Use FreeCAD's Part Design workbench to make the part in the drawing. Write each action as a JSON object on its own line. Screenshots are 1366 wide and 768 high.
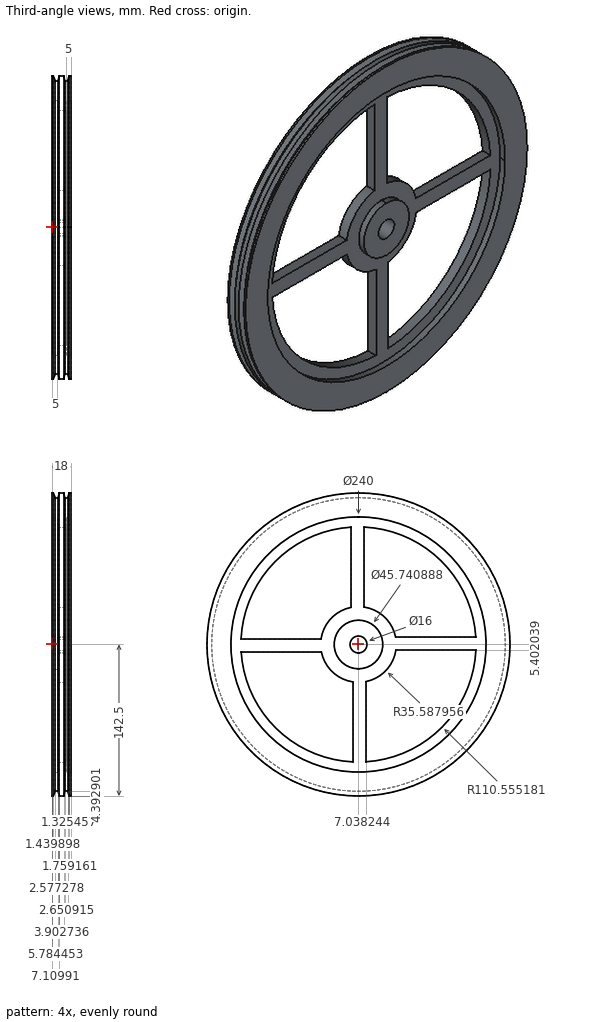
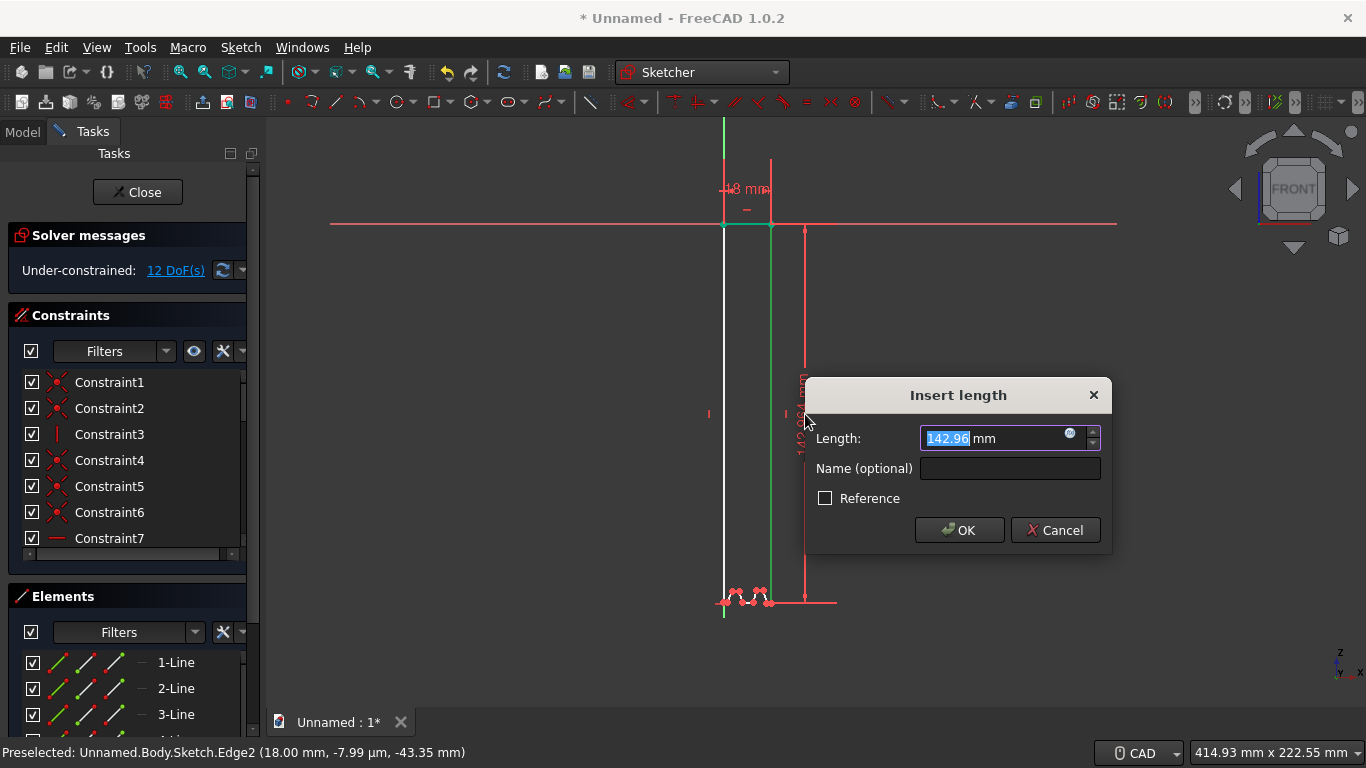
{"action": "type", "text": "142.5"}
{"action": "key", "text": "Return"}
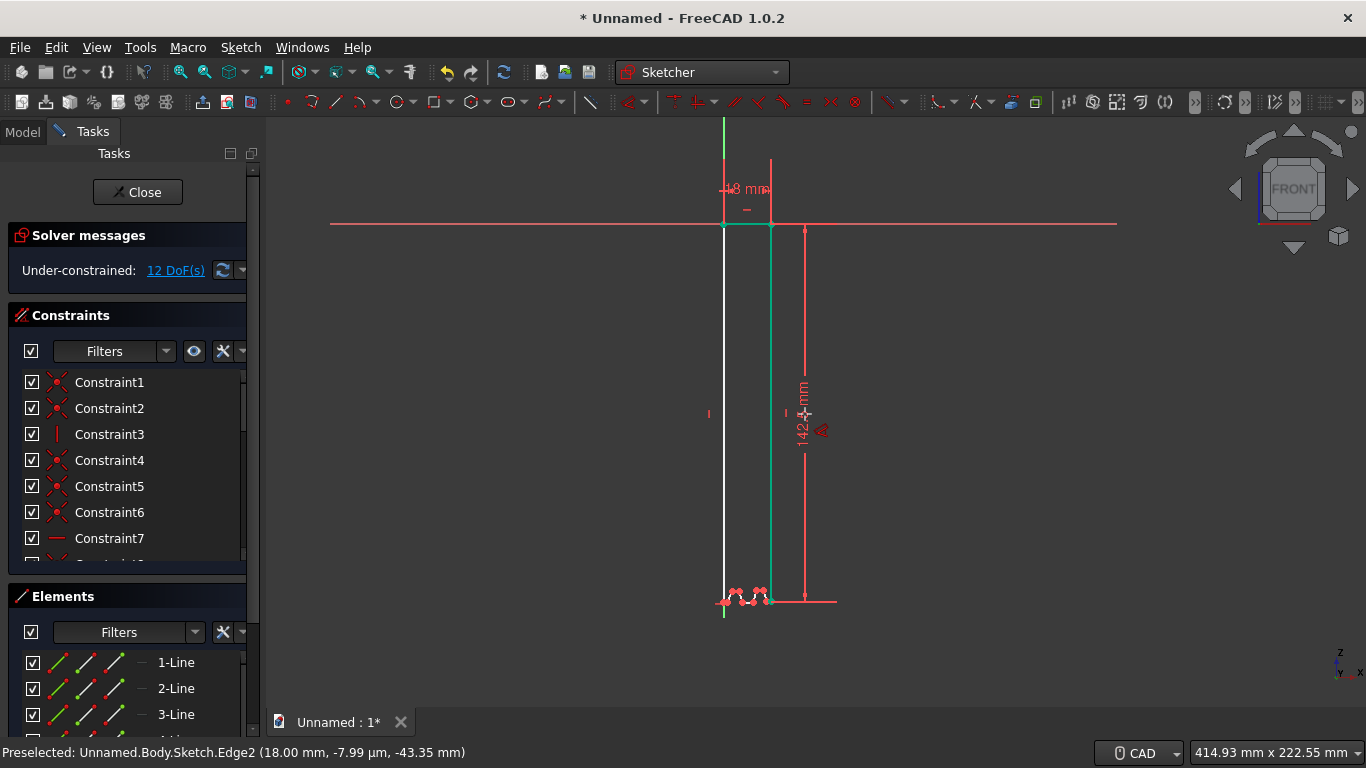
{"action": "left_click", "coordinate": [724, 489]}
{"action": "left_click", "coordinate": [690, 413]}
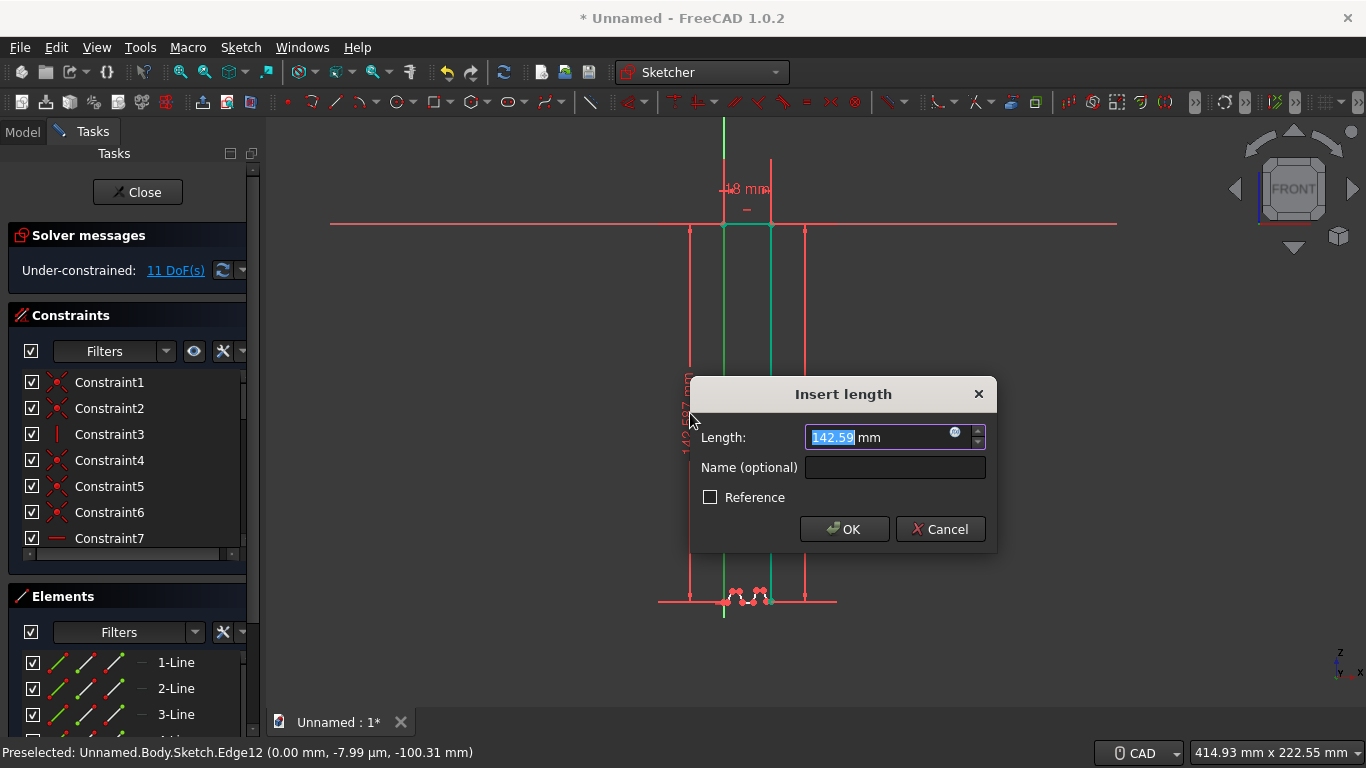
{"action": "type", "text": "142.5"}
{"action": "key", "text": "Return"}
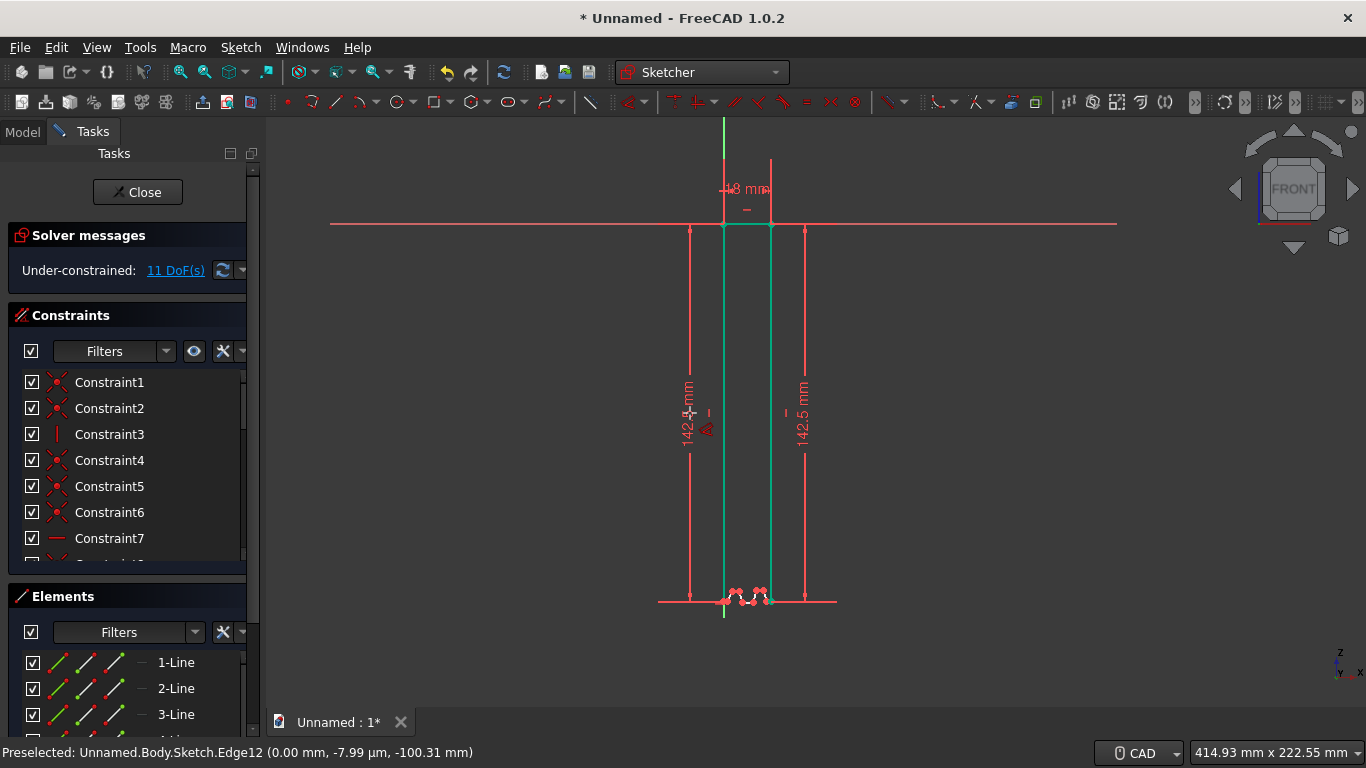
{"action": "left_click", "coordinate": [753, 603]}
{"action": "left_click", "coordinate": [690, 326]}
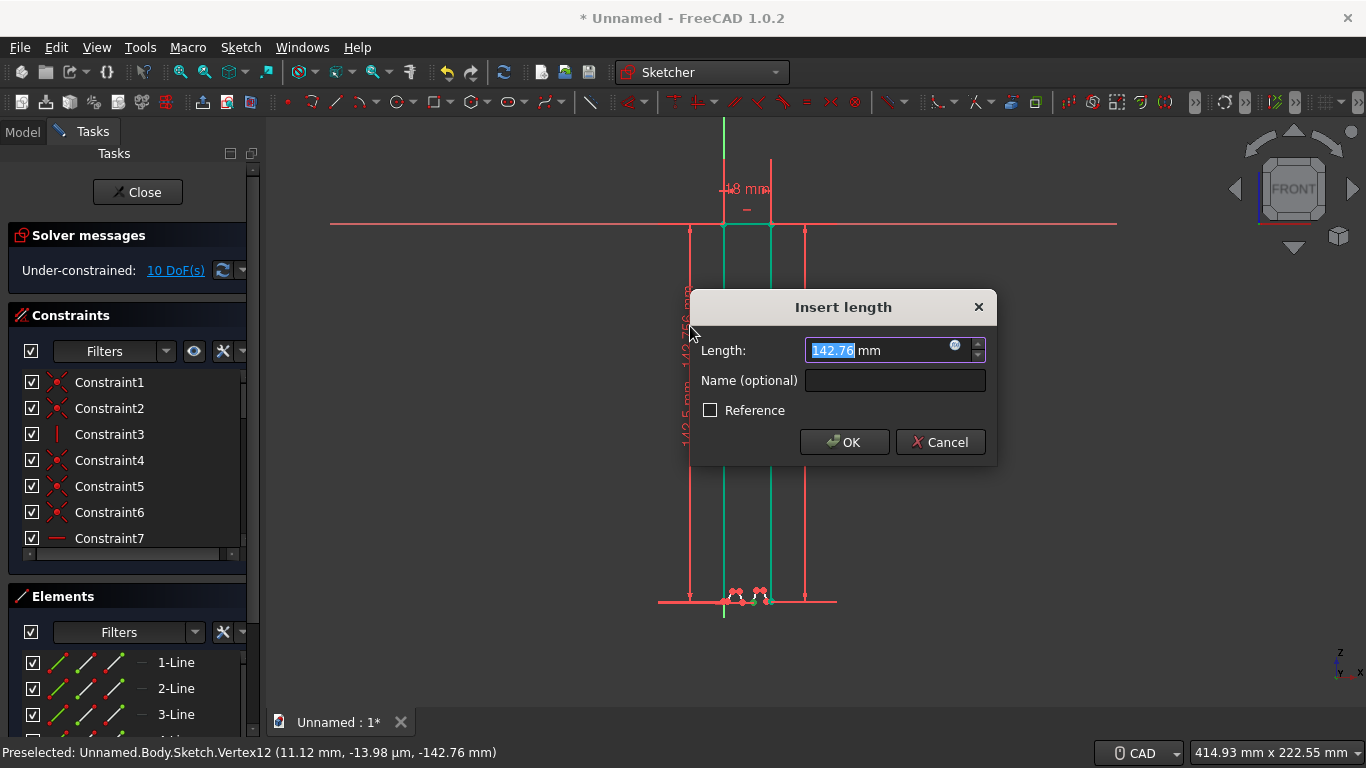
{"action": "type", "text": "142.5"}
{"action": "key", "text": "Return"}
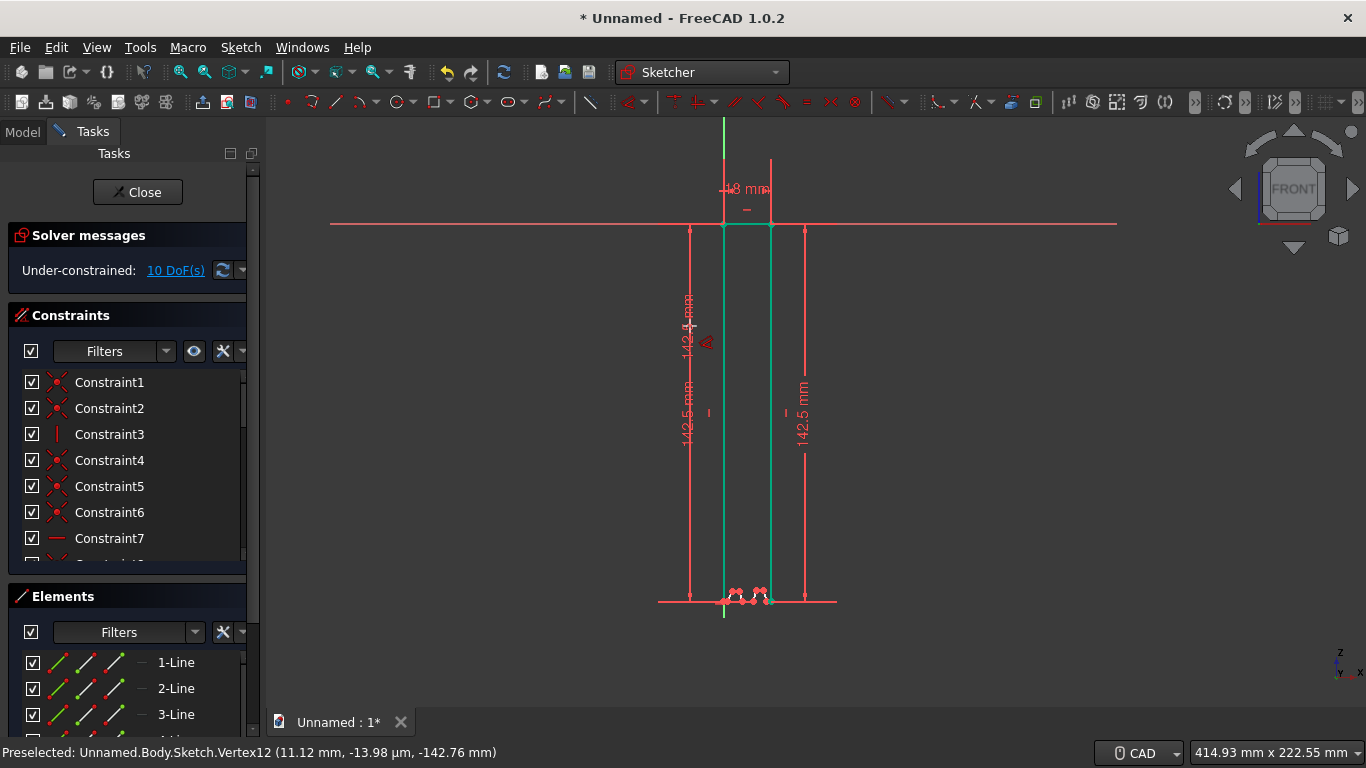
{"action": "scroll", "coordinate": [769, 602], "scroll_direction": "up", "scroll_amount": 11}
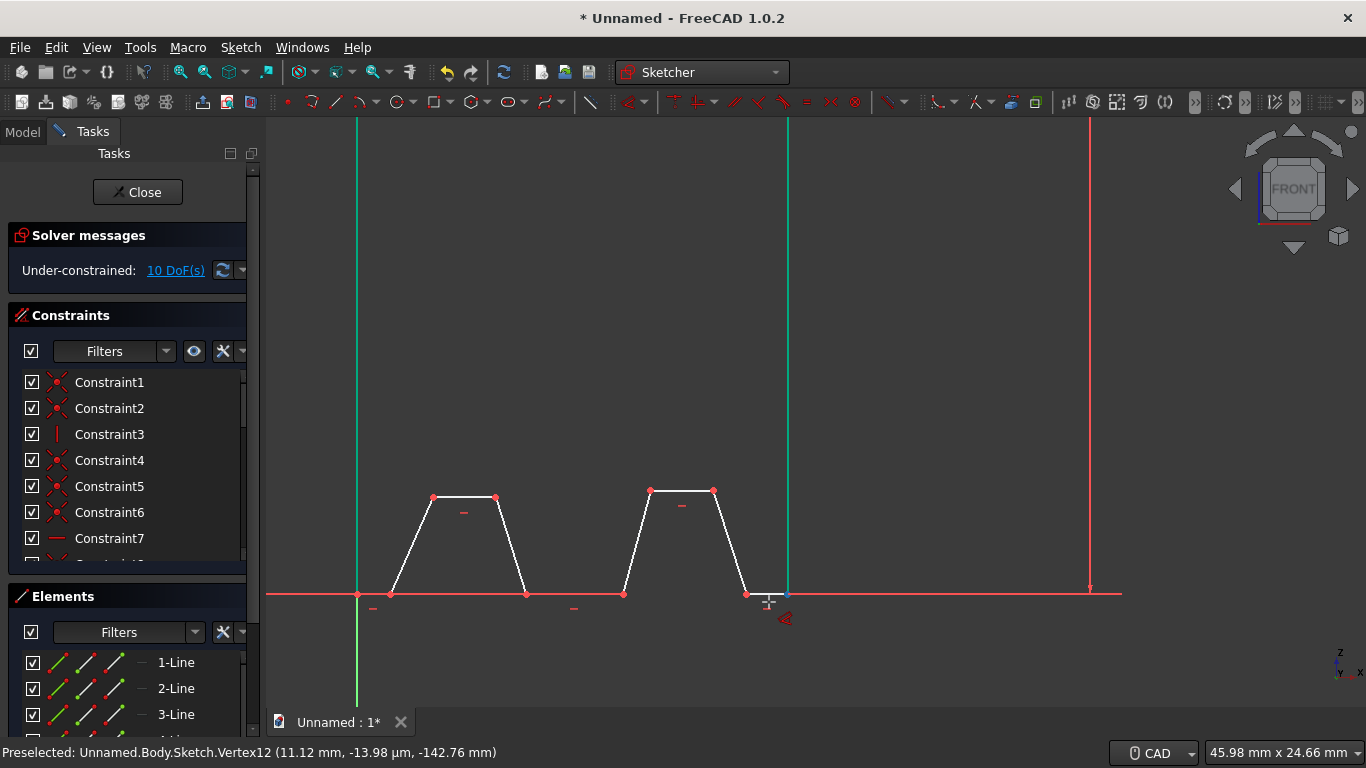
{"action": "left_click", "coordinate": [767, 594]}
{"action": "left_click", "coordinate": [767, 628]}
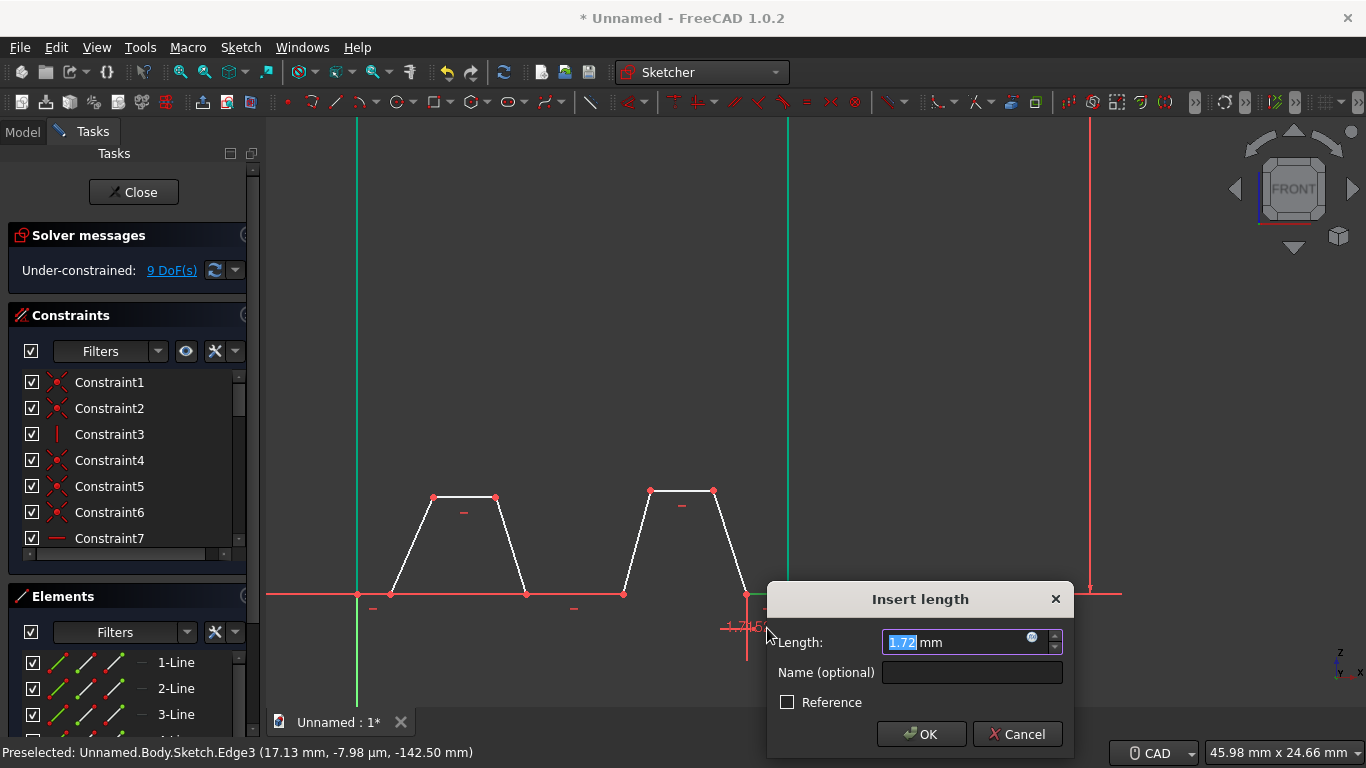
{"action": "type", "text": "1.759161"}
{"action": "key", "text": "Return"}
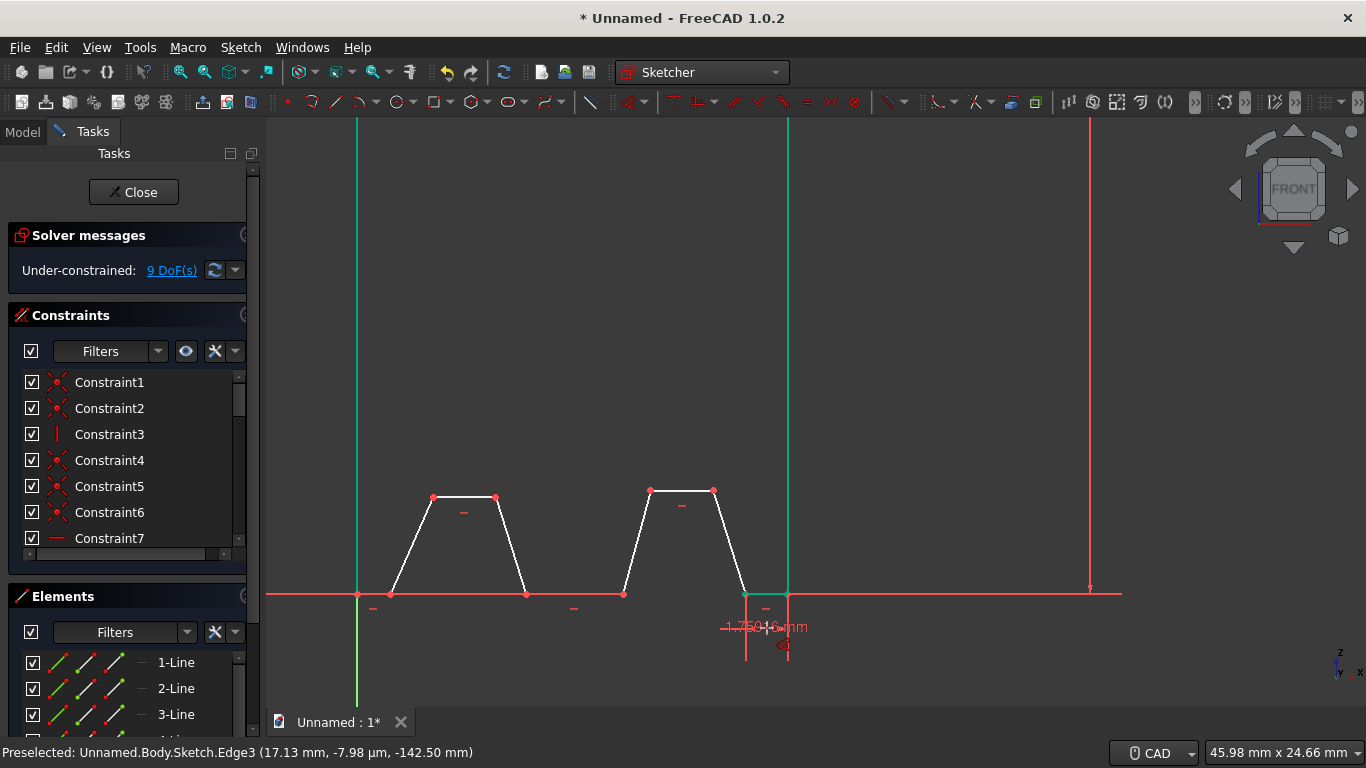
{"action": "left_click", "coordinate": [695, 491]}
{"action": "left_click", "coordinate": [682, 525]}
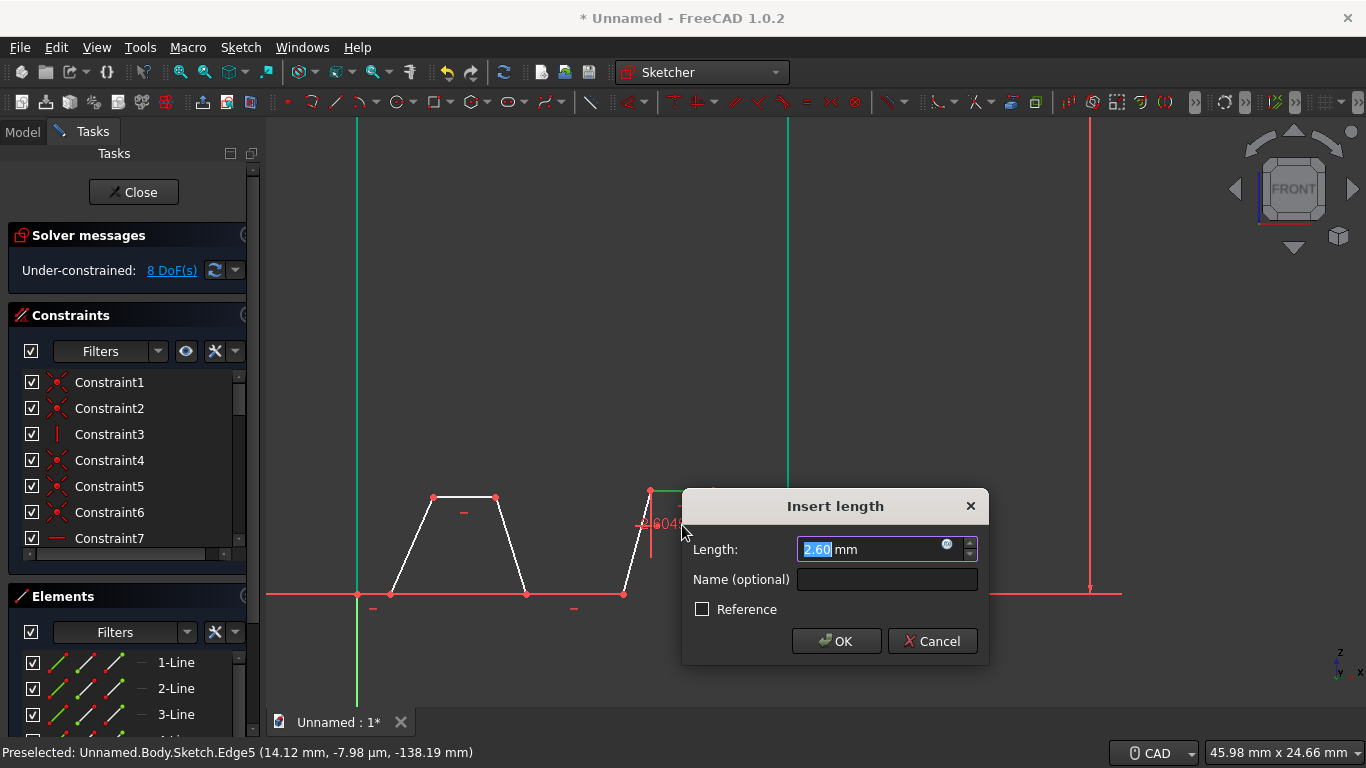
{"action": "type", "text": "2.650915"}
{"action": "key", "text": "Return"}